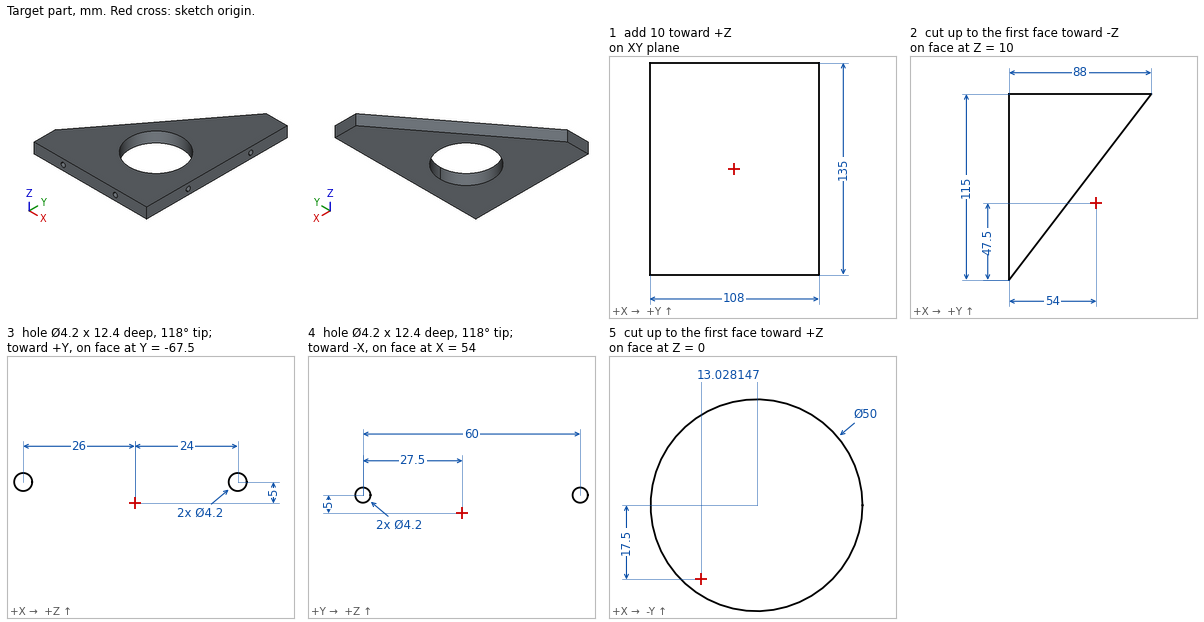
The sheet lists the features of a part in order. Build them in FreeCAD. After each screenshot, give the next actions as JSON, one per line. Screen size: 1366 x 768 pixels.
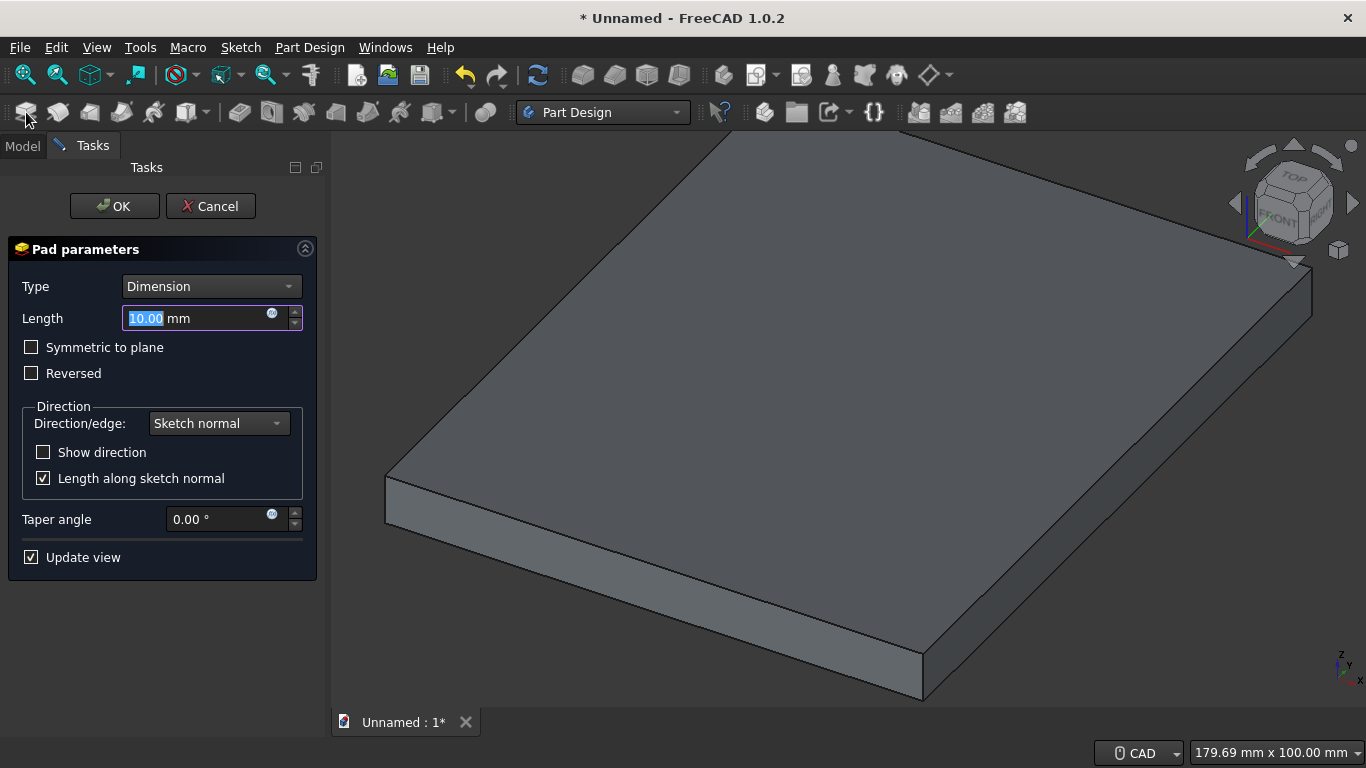
{"action": "type", "text": "10"}
{"action": "key", "text": "Tab"}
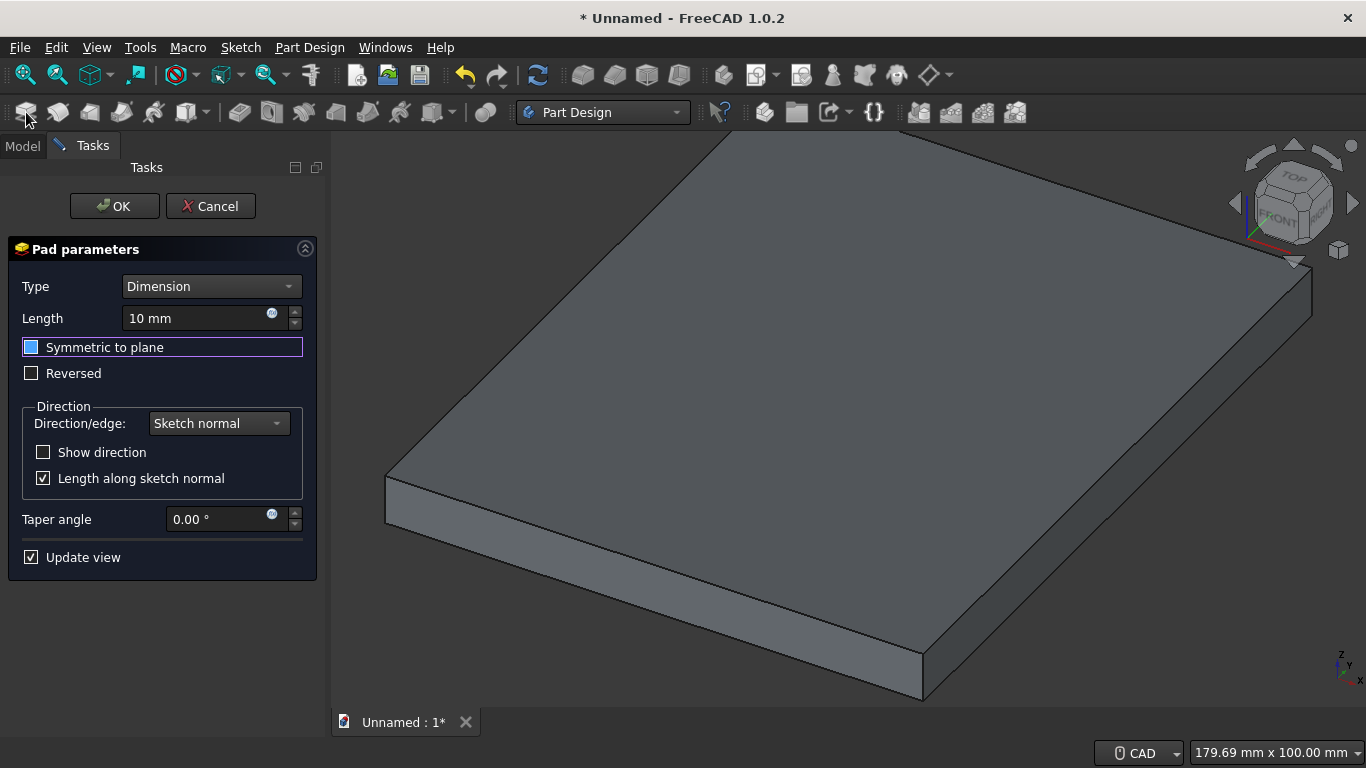
{"action": "left_click", "coordinate": [115, 206]}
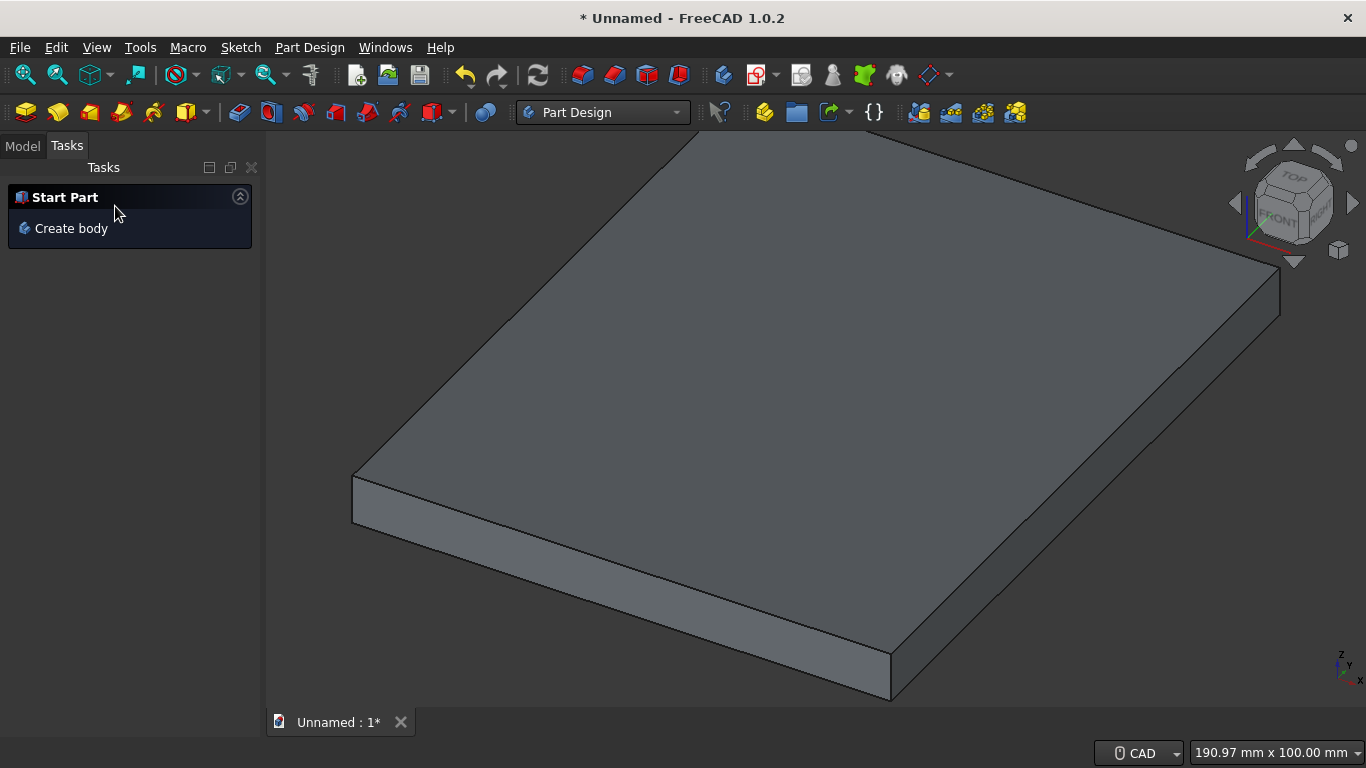
{"action": "key", "text": "v f"}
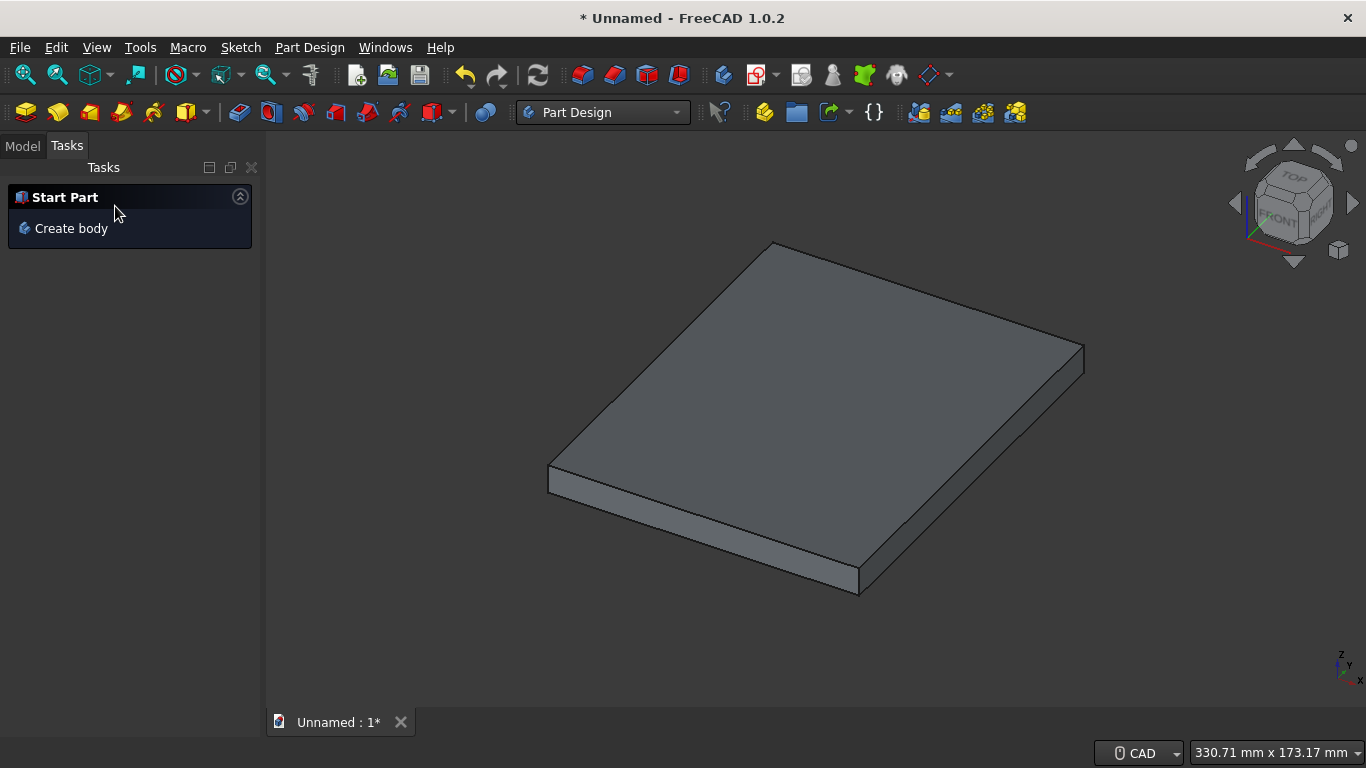
{"action": "left_click", "coordinate": [816, 404]}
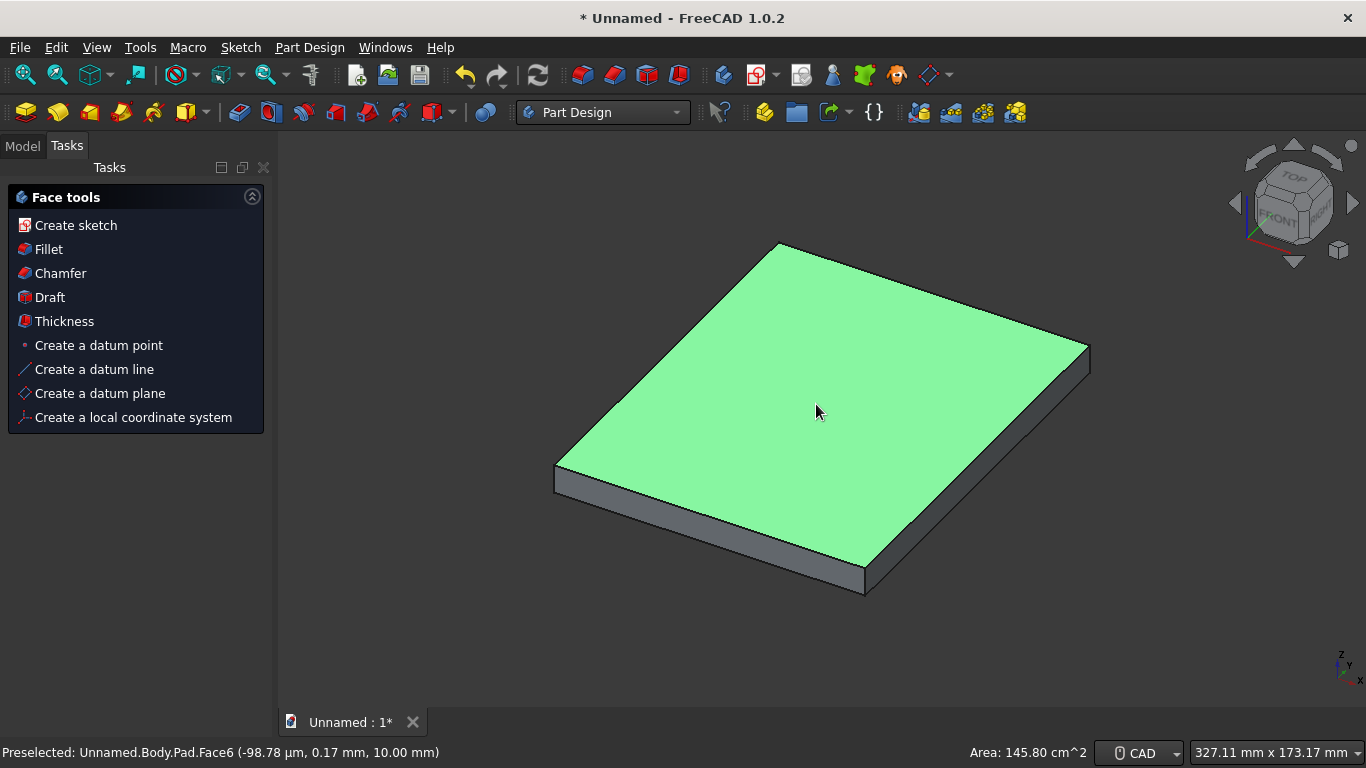
{"action": "left_click", "coordinate": [756, 76]}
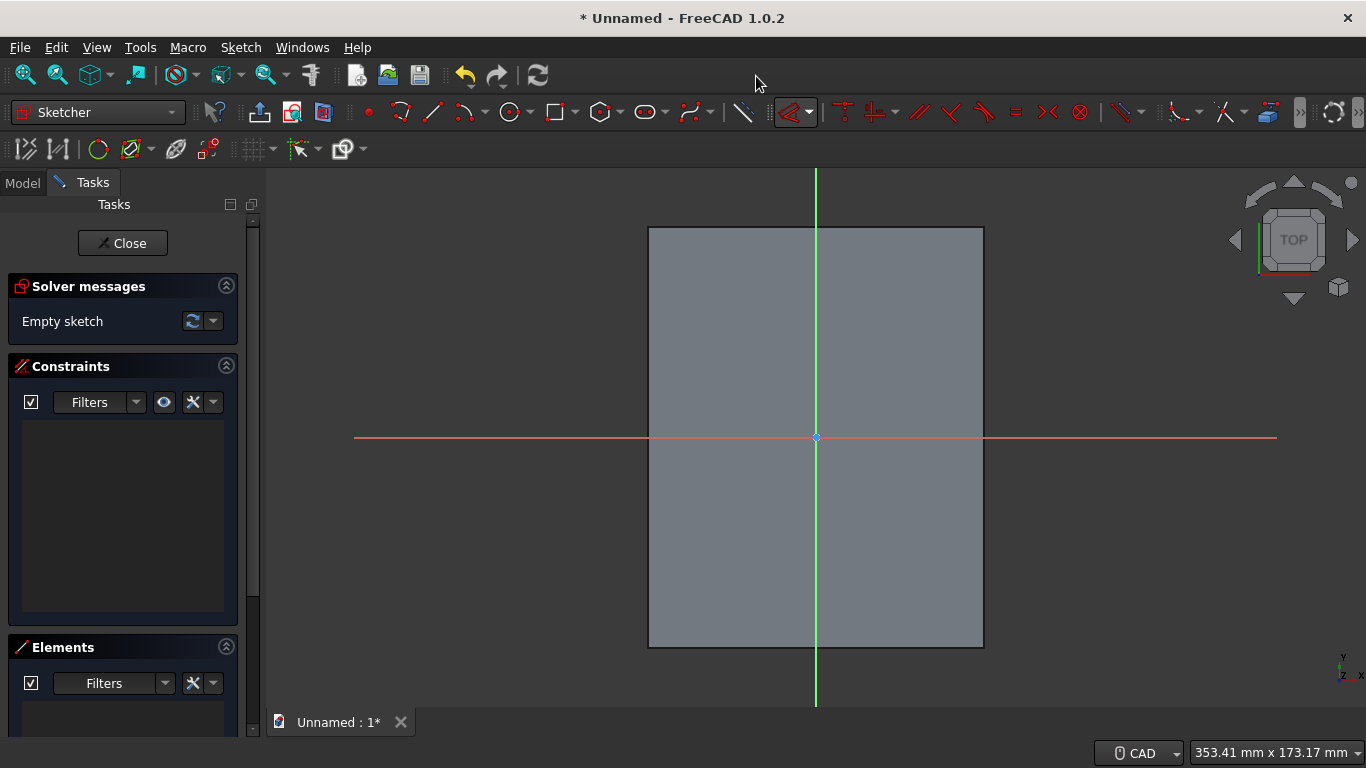
{"action": "key", "text": "g m"}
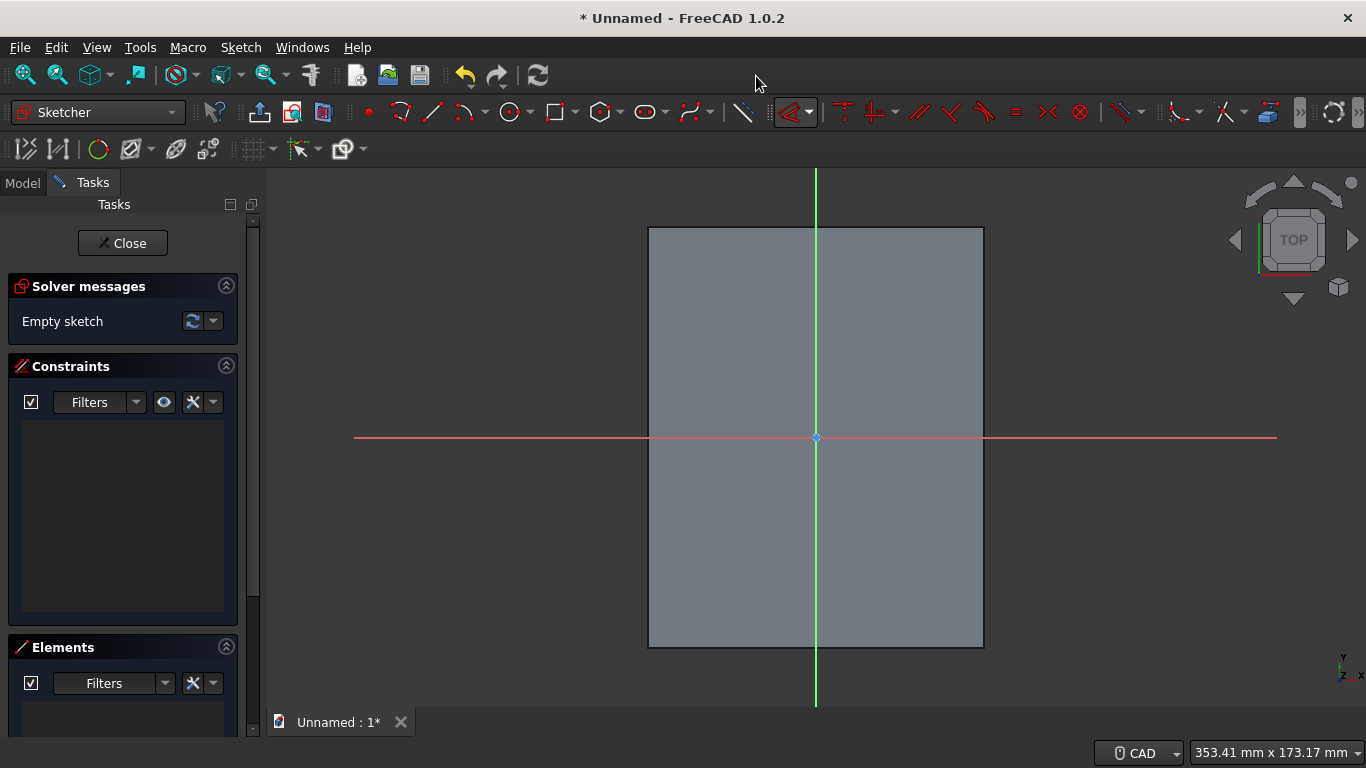
{"action": "left_click", "coordinate": [648, 585]}
{"action": "left_click", "coordinate": [922, 227]}
{"action": "left_click", "coordinate": [648, 227]}
{"action": "left_click", "coordinate": [648, 586]}
{"action": "key", "text": "Escape"}
{"action": "key", "text": "Escape"}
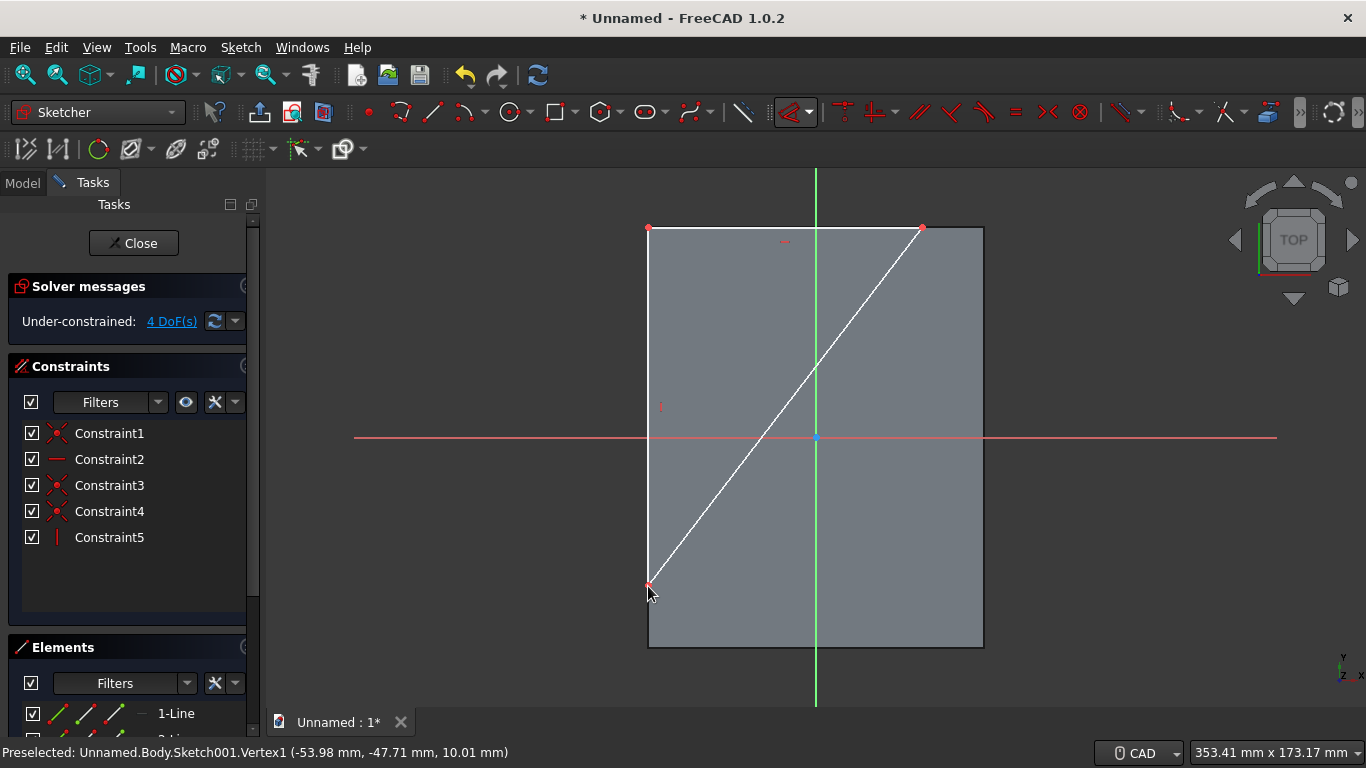
{"action": "left_click", "coordinate": [790, 112]}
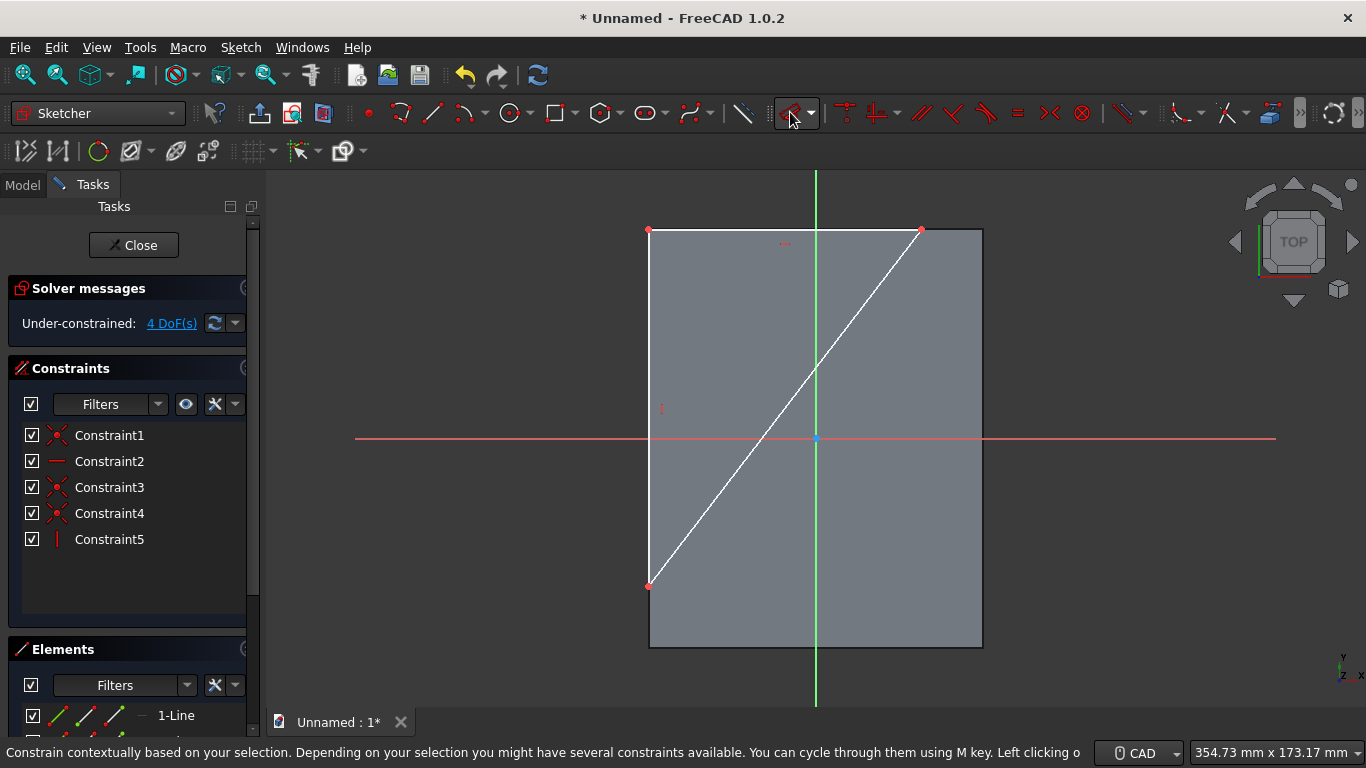
{"action": "left_click", "coordinate": [840, 230]}
{"action": "left_click", "coordinate": [785, 264]}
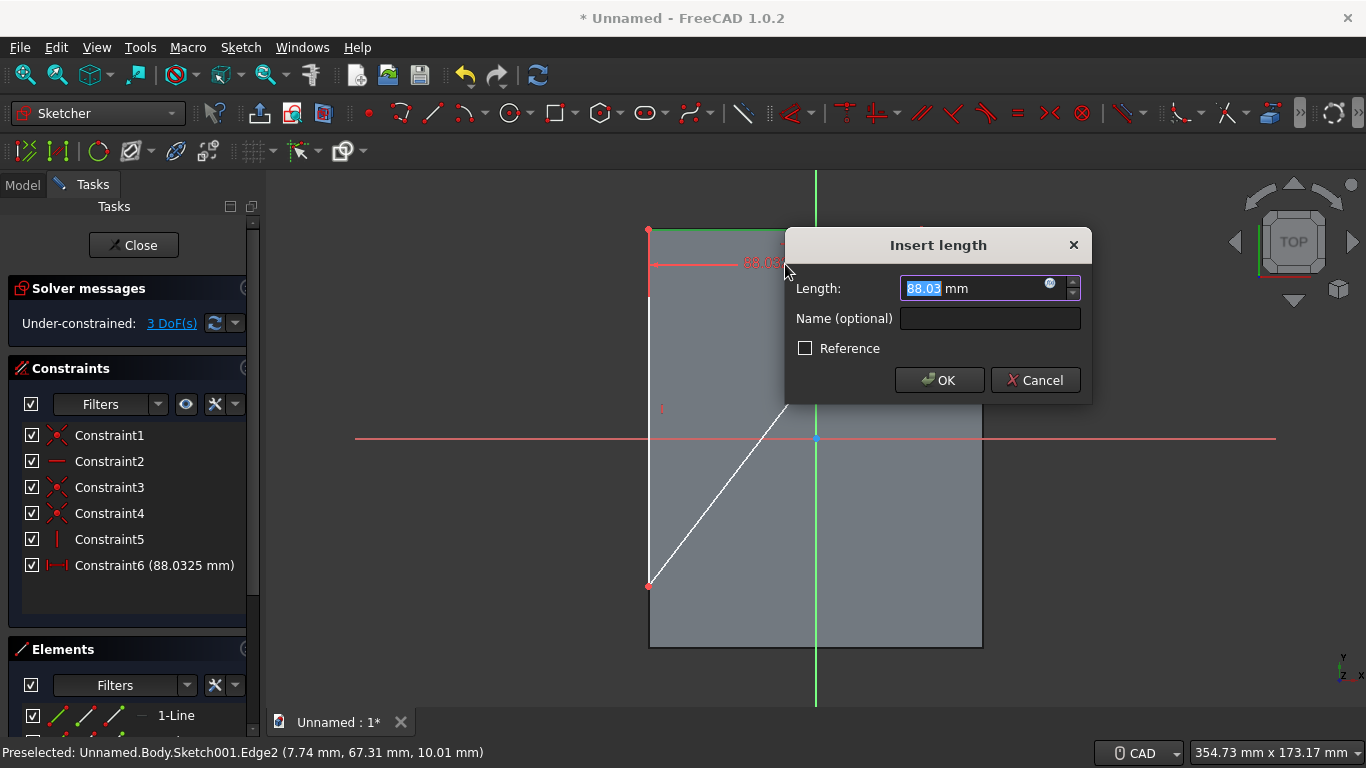
{"action": "type", "text": "88"}
{"action": "key", "text": "Return"}